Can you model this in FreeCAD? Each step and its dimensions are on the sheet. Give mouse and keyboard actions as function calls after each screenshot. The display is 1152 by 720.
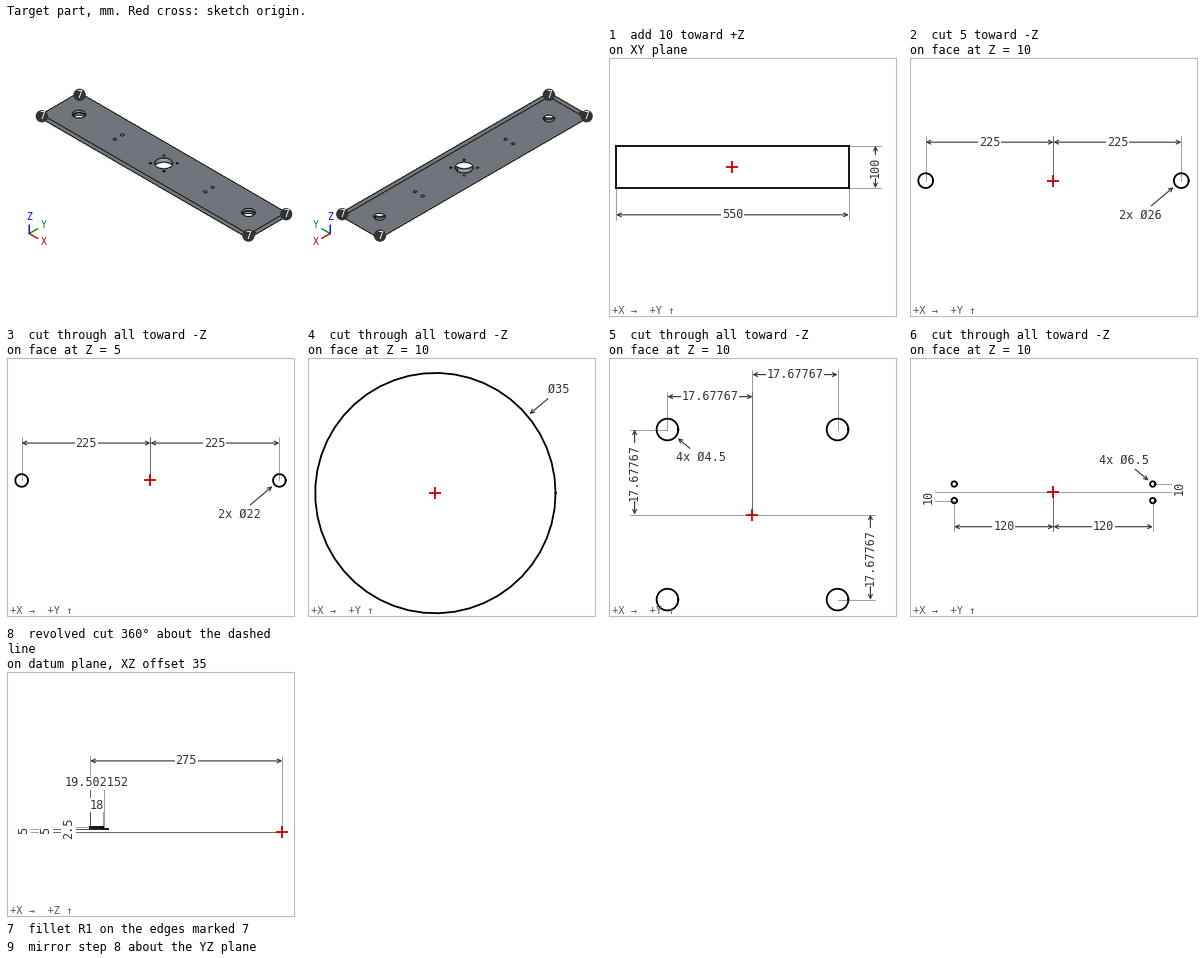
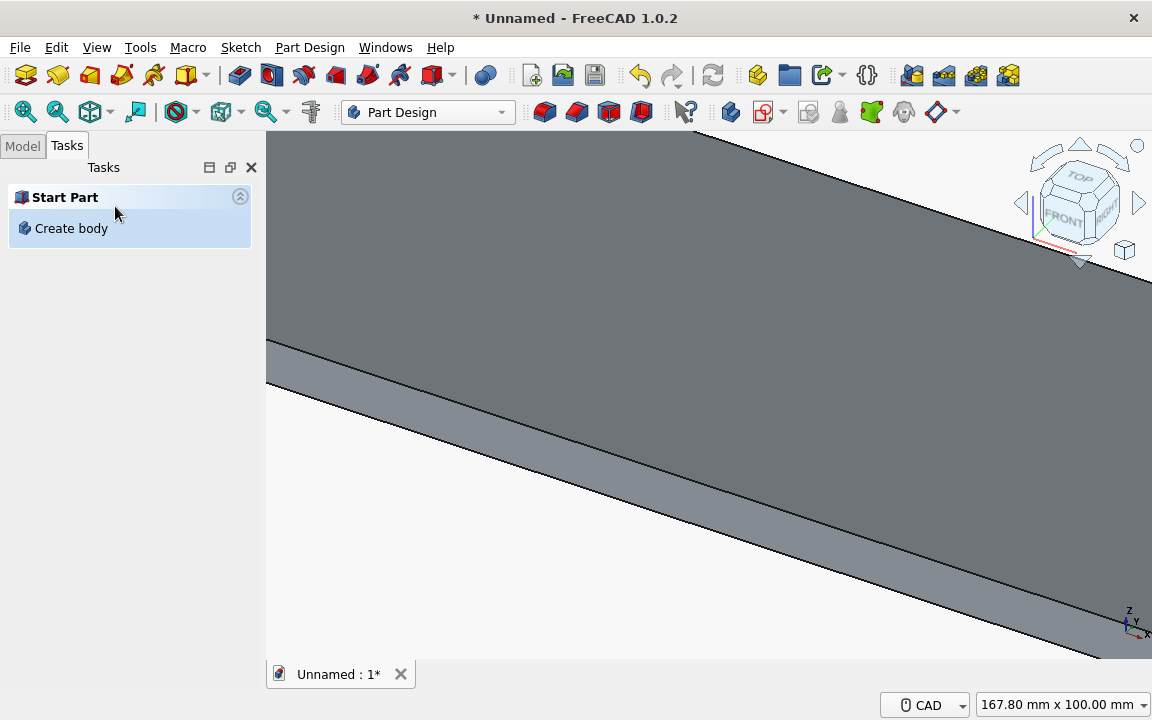
click(26, 112)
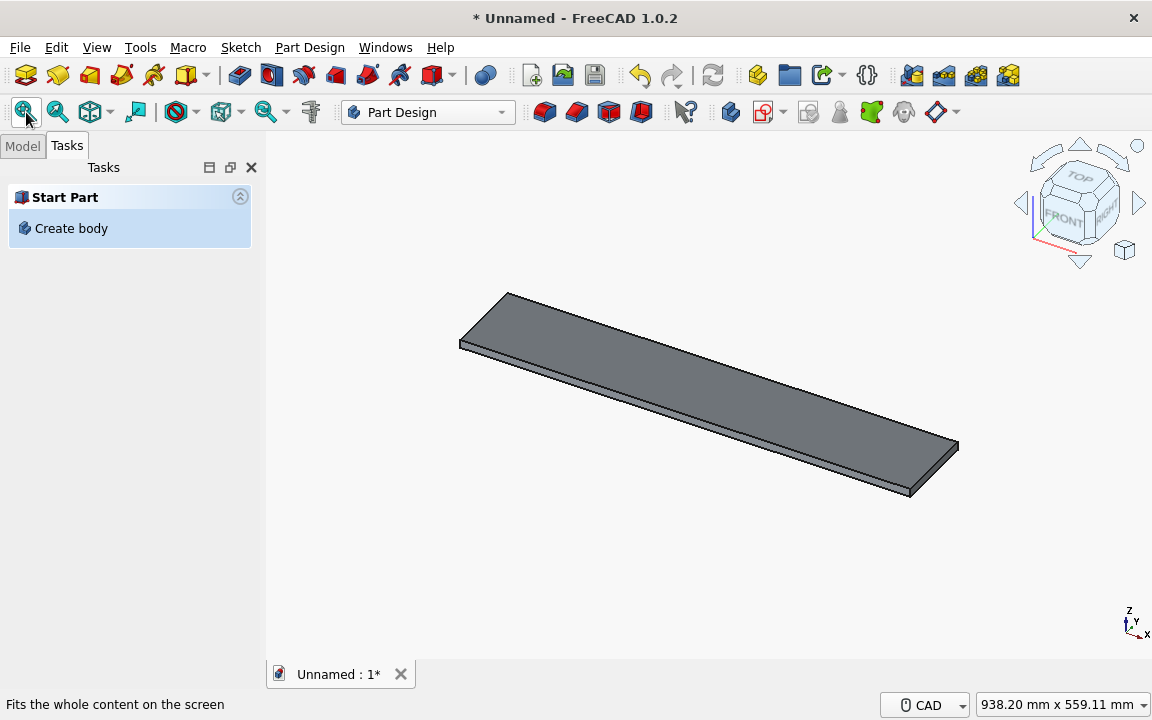
click(838, 433)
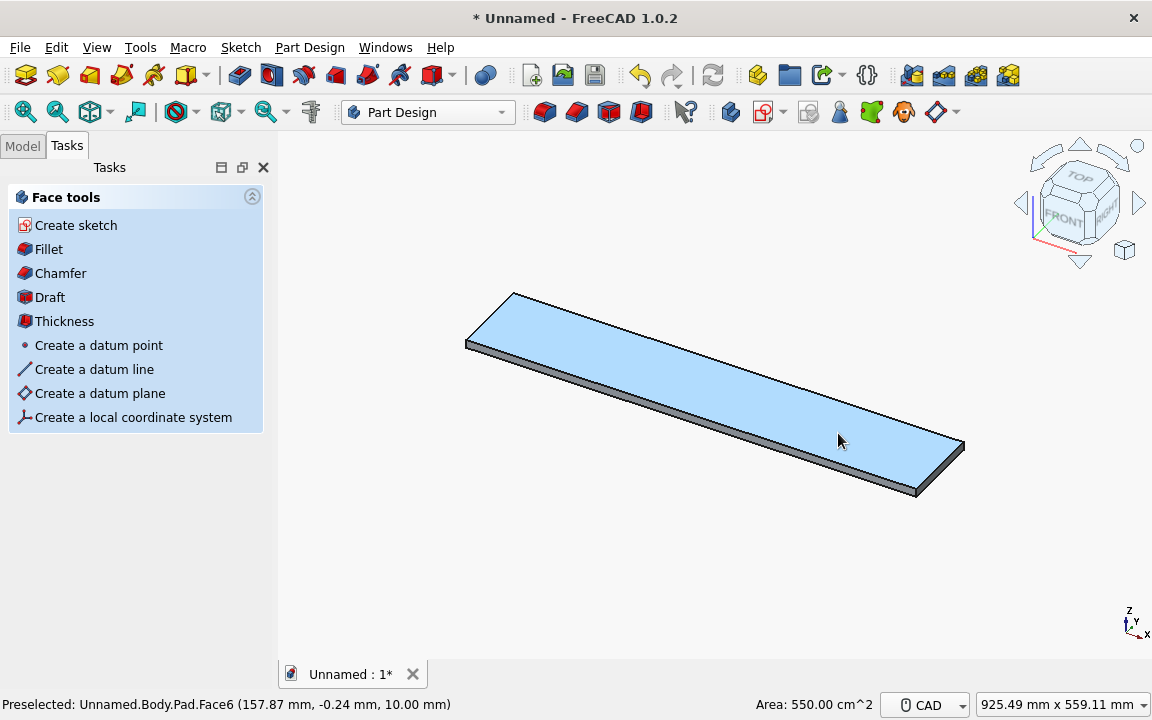
click(764, 112)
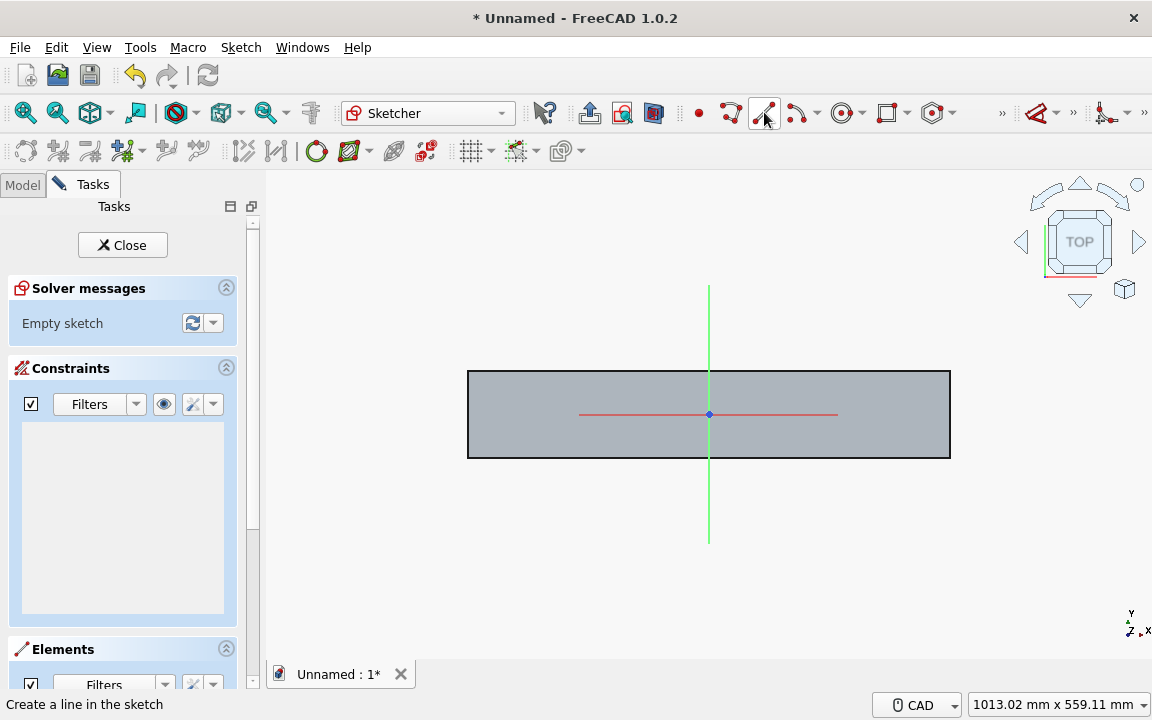
click(842, 114)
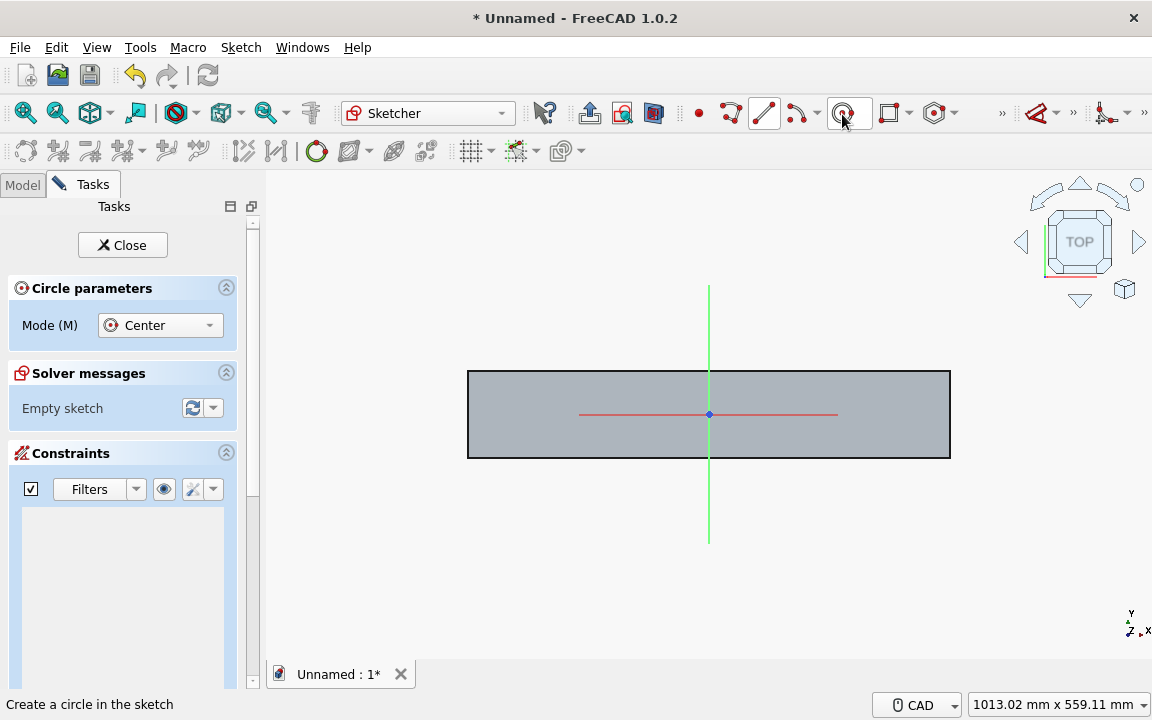
scroll(906, 414, up, 4)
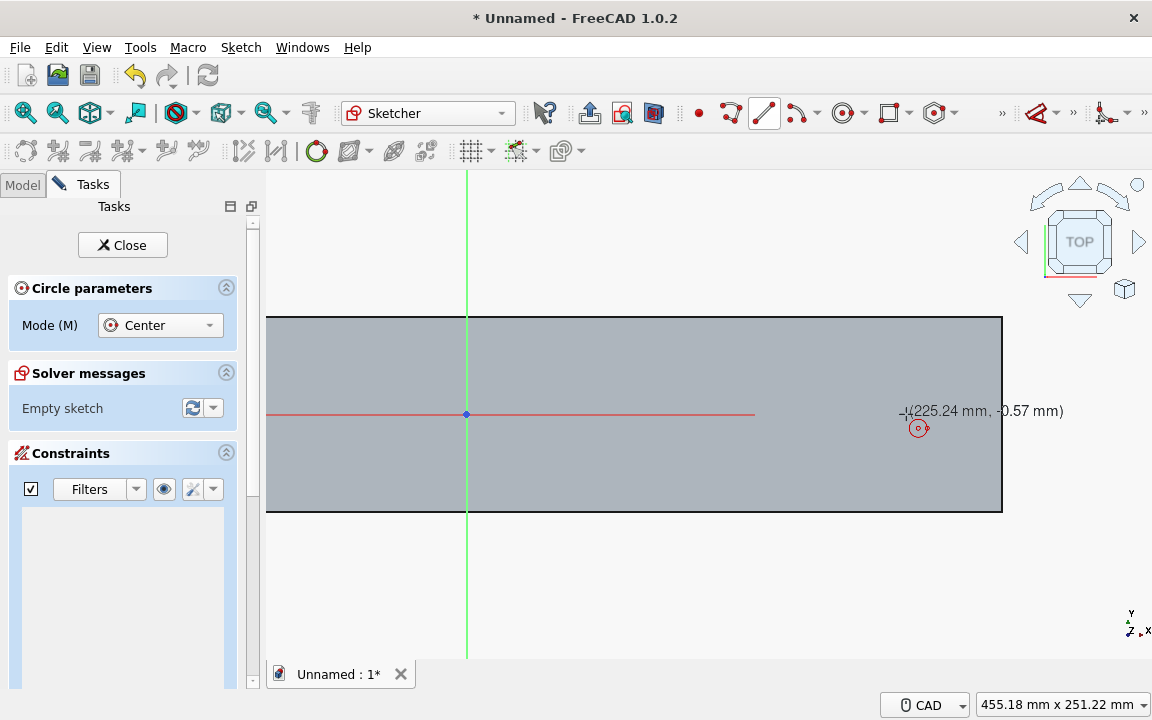
click(905, 414)
move(923, 397)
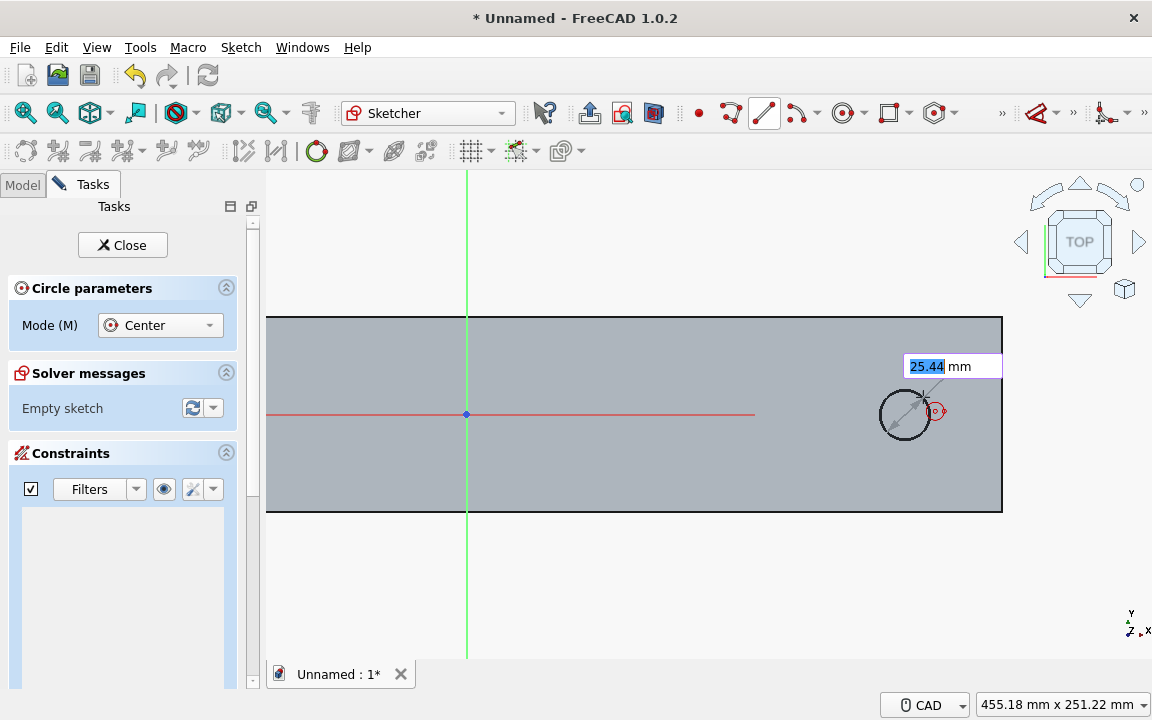
text(26)
key(Return)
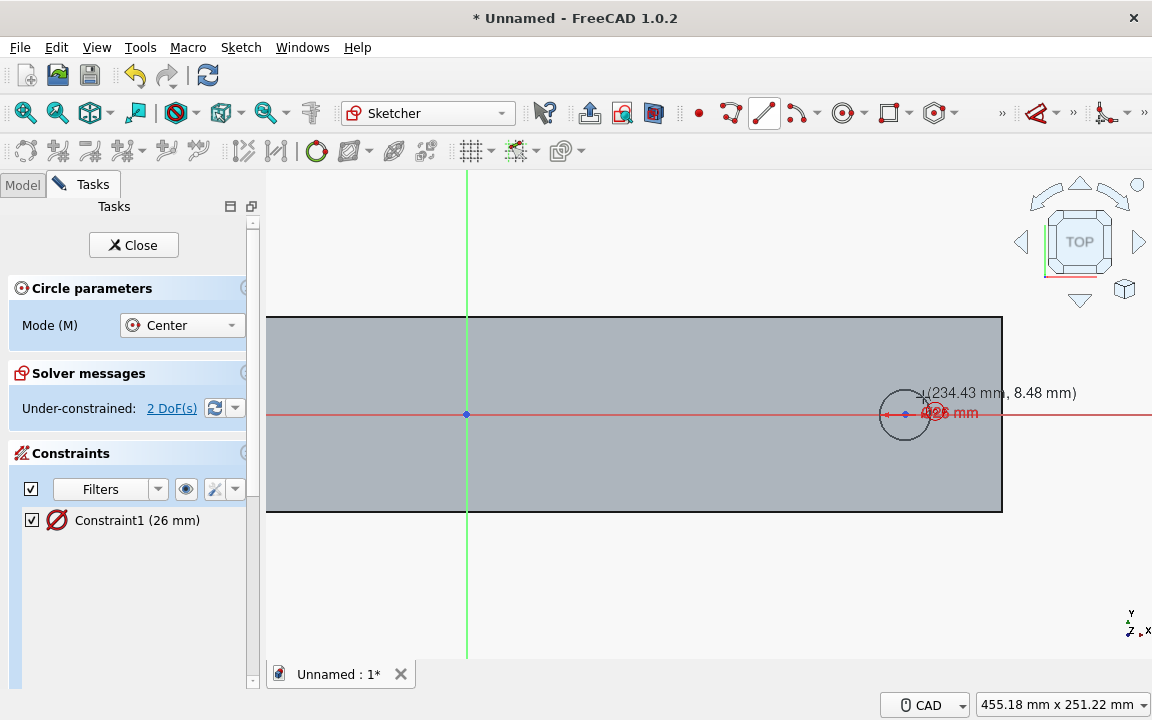
scroll(852, 414, down, 3)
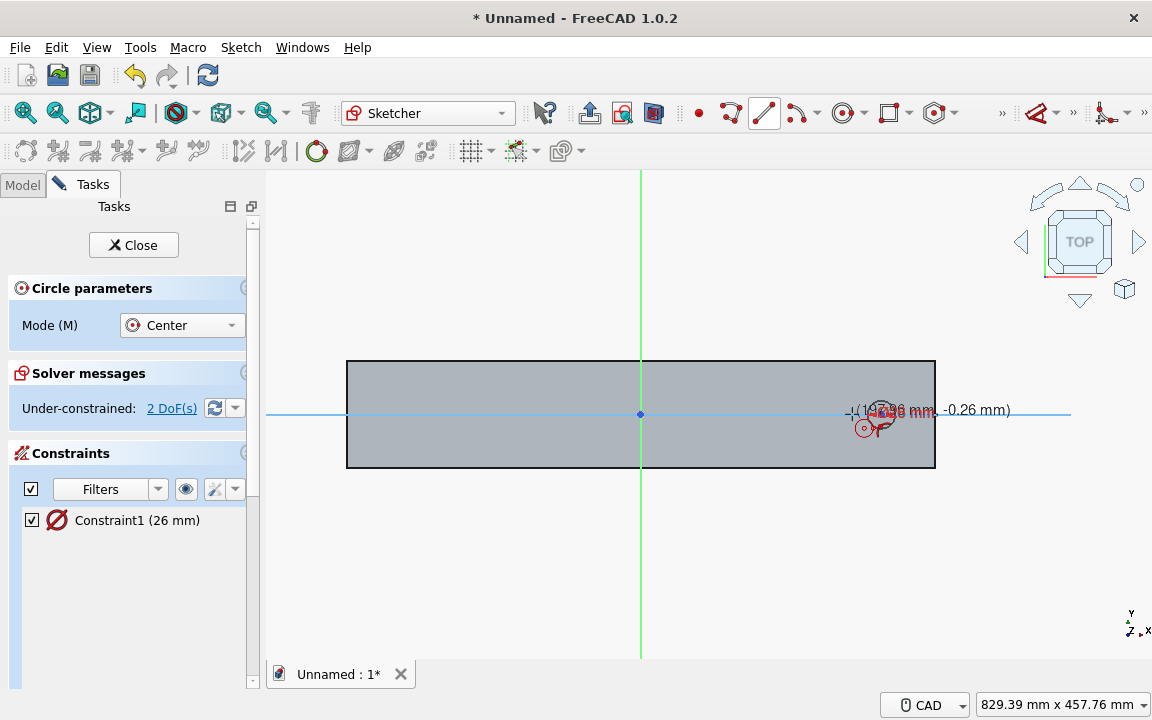
scroll(400, 414, up, 3)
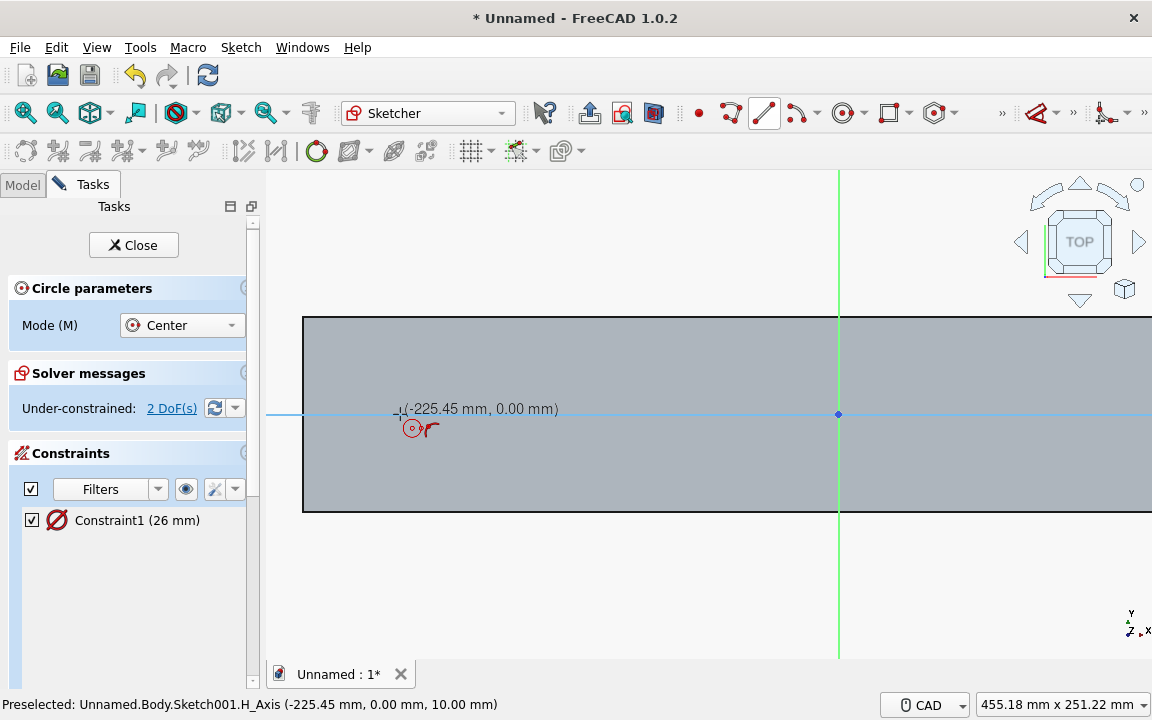
click(401, 414)
move(419, 397)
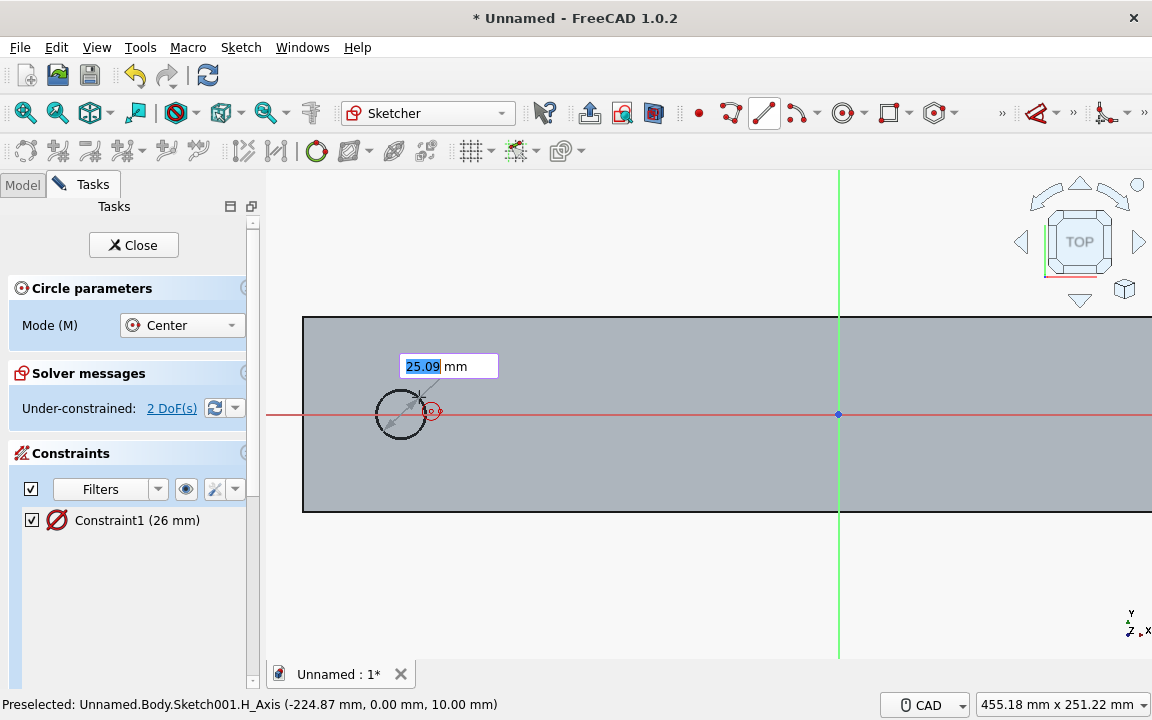
text(26)
key(Return)
key(Escape)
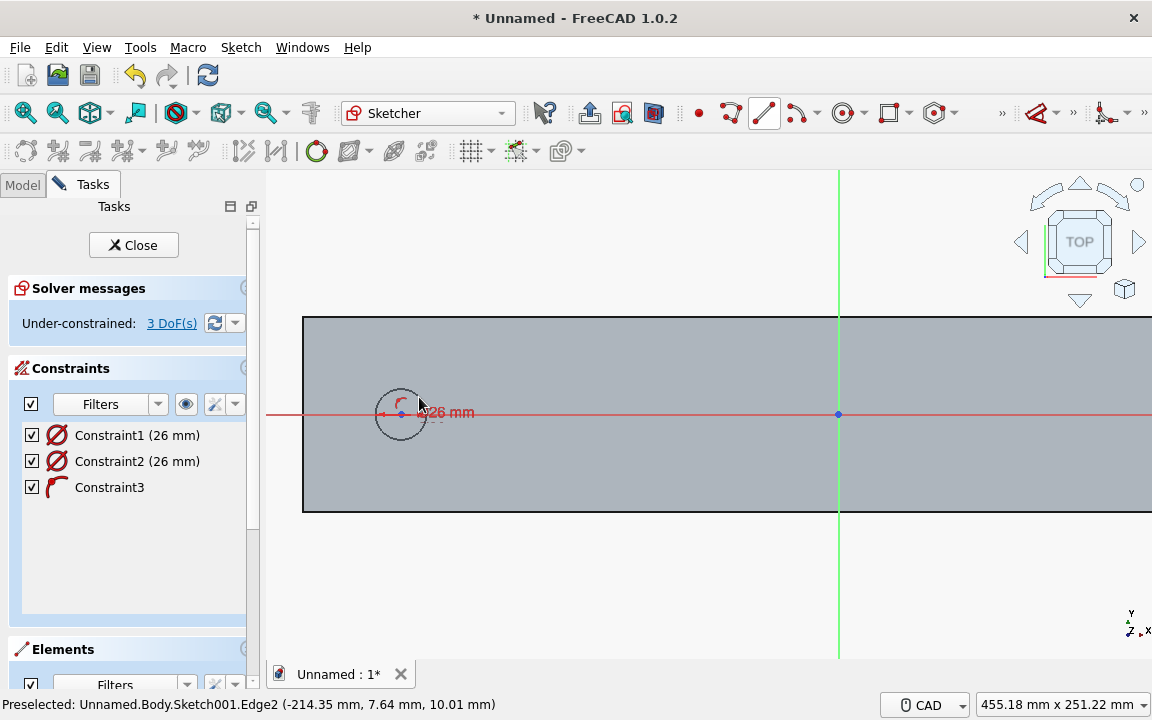
scroll(399, 414, down, 3)